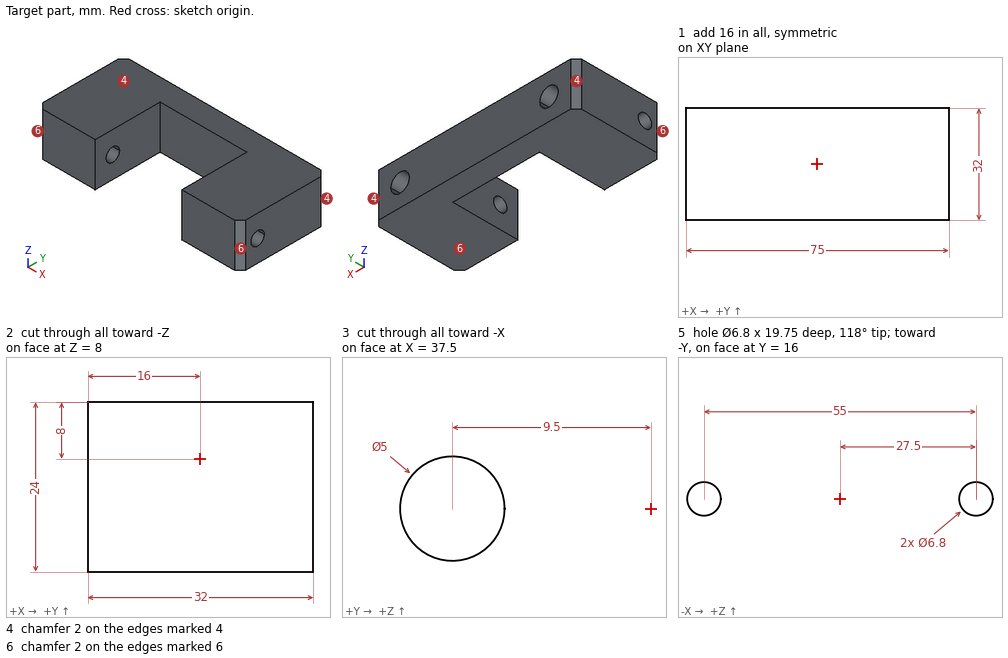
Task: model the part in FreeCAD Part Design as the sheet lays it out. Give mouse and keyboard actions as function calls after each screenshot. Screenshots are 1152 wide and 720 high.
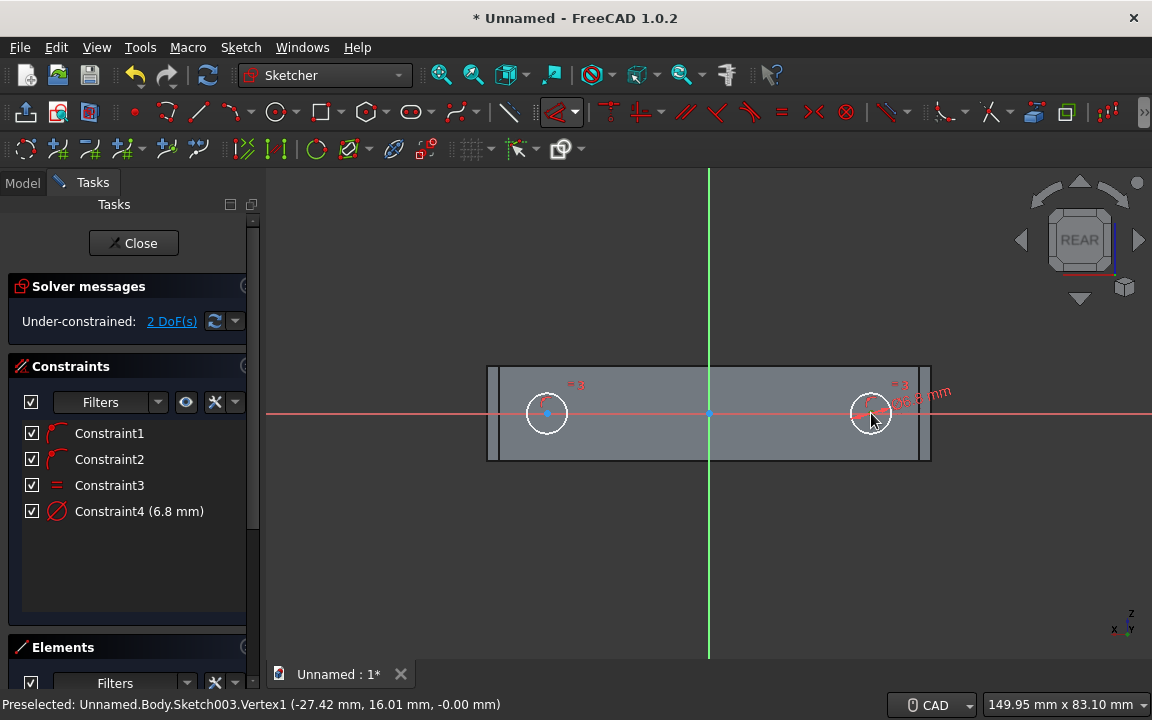
click(547, 413)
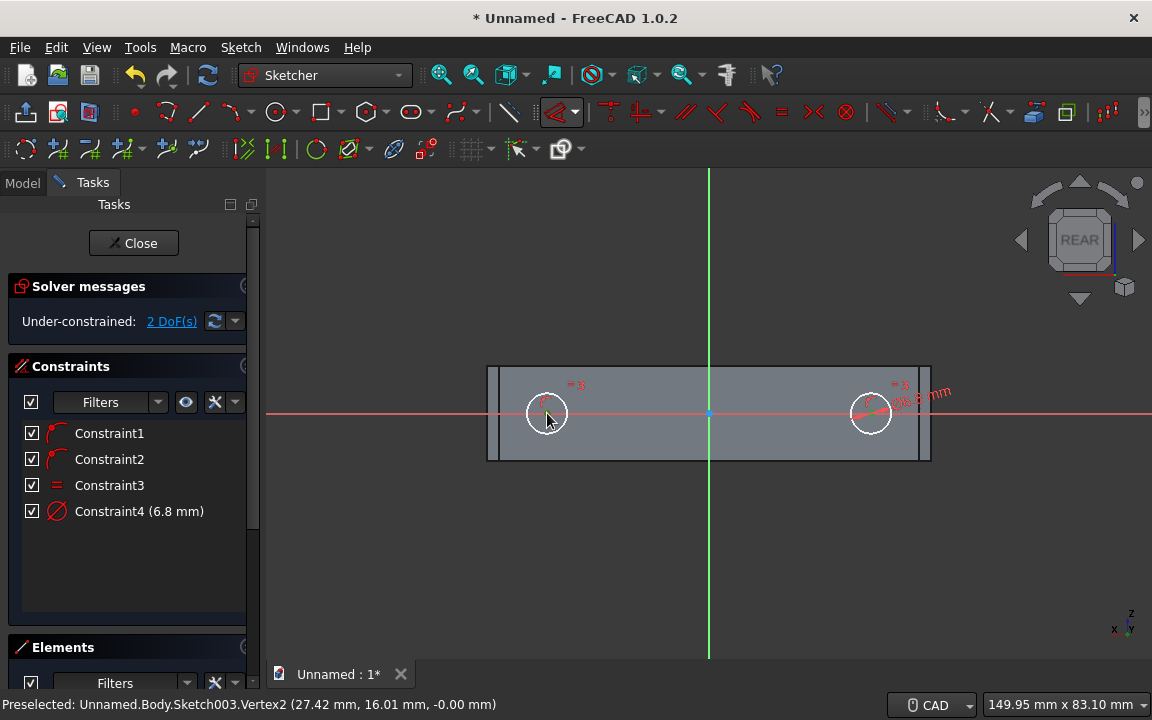
key(l)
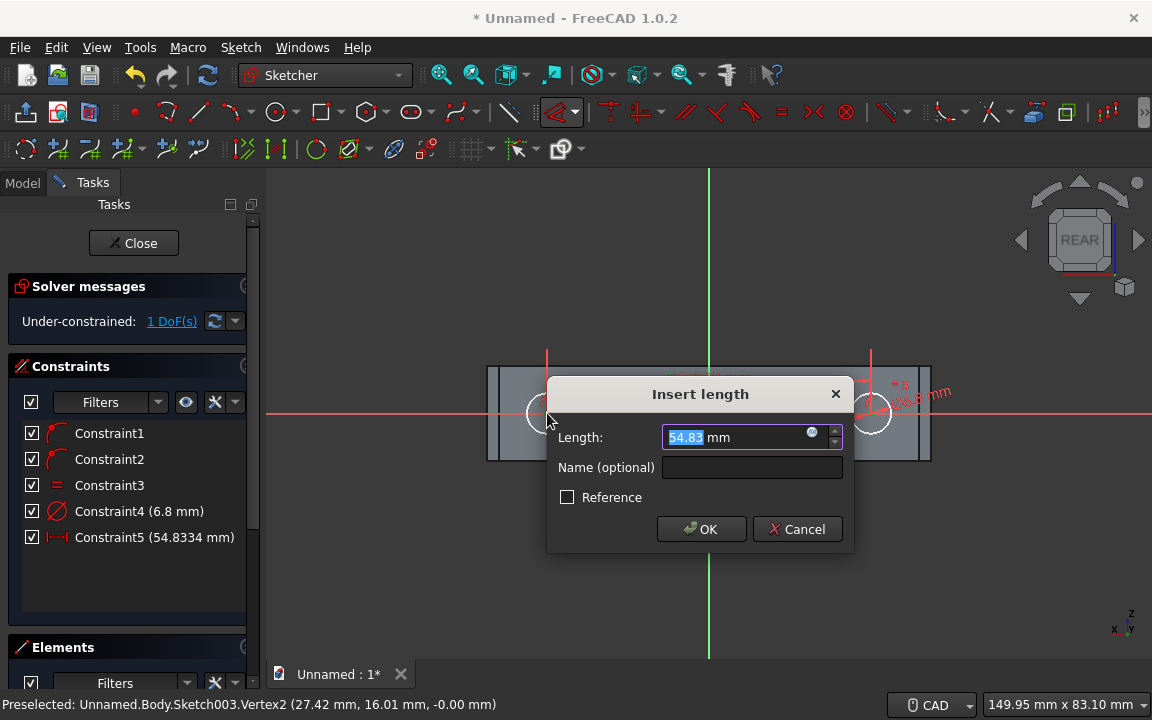
text(55)
key(Return)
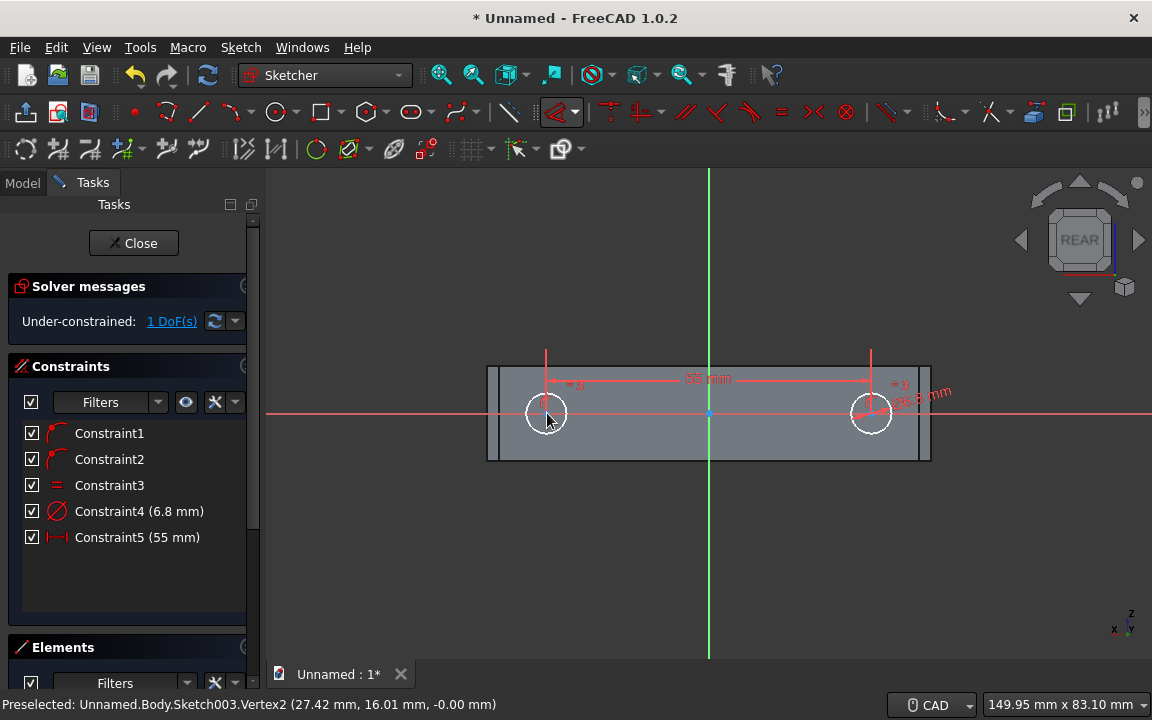
click(871, 413)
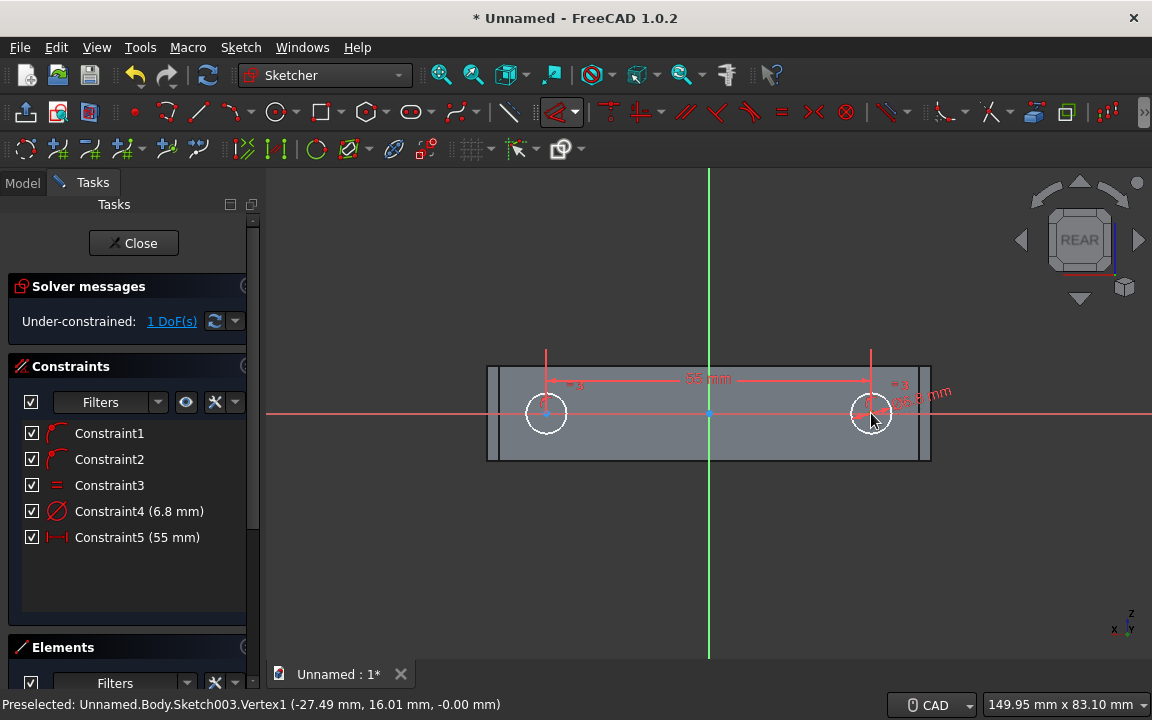
click(578, 112)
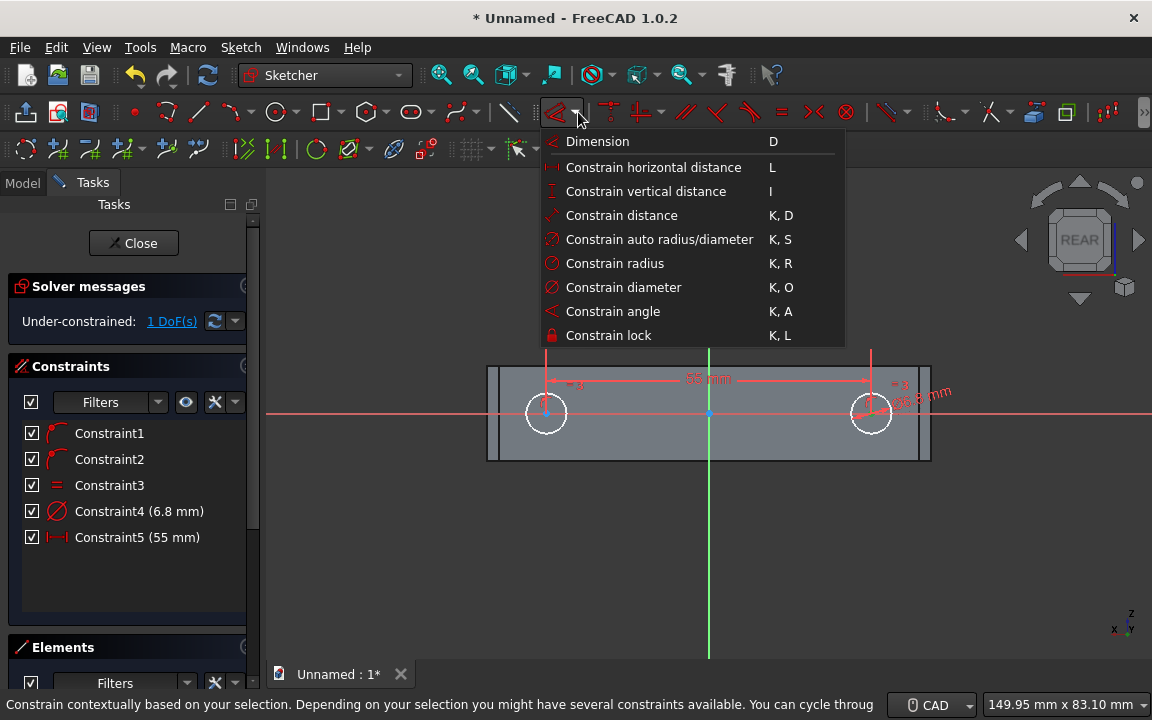
click(693, 167)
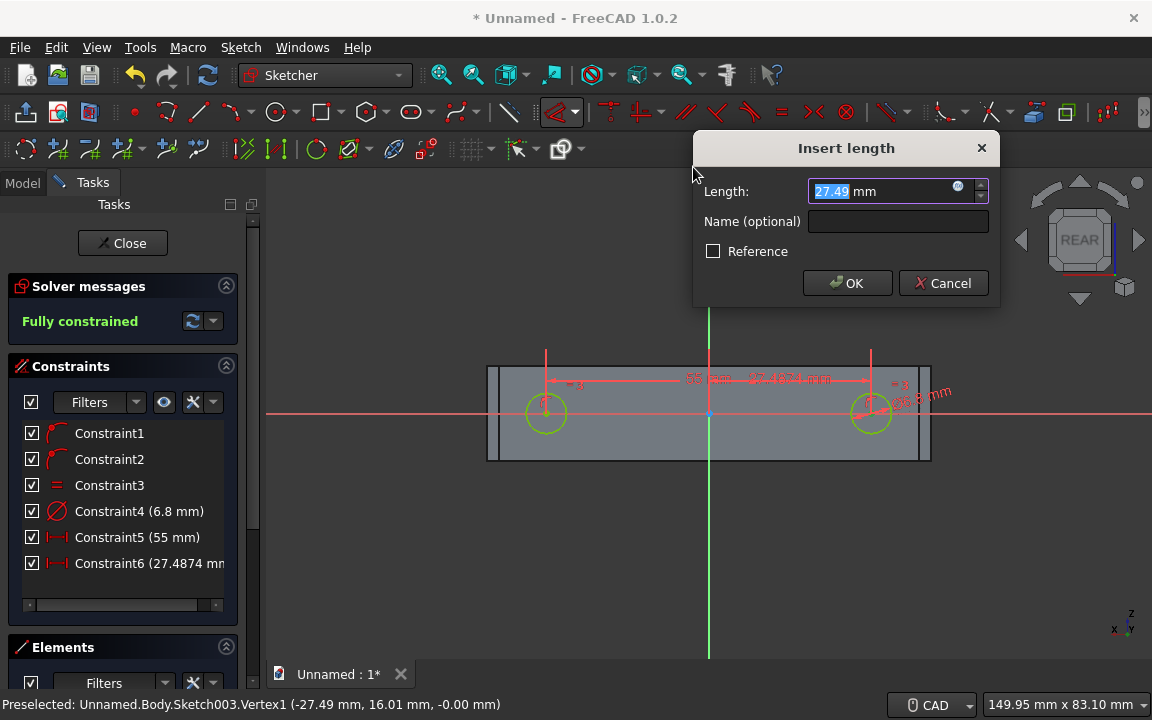
text(27.5)
key(Return)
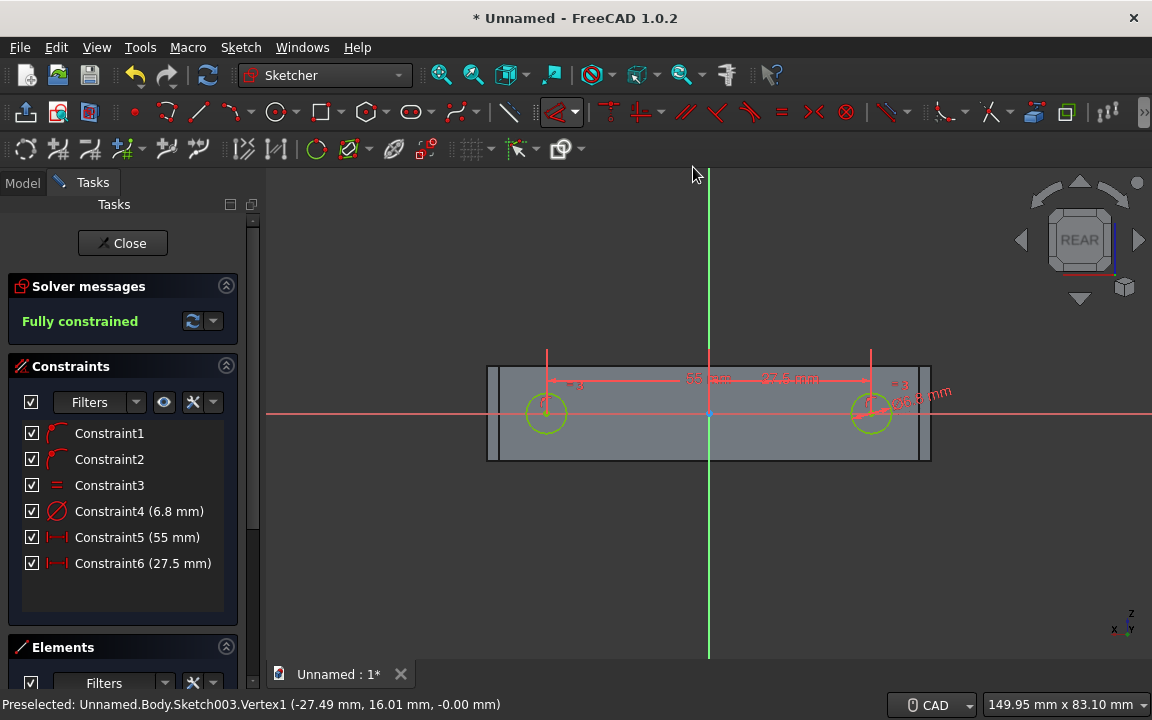
click(123, 243)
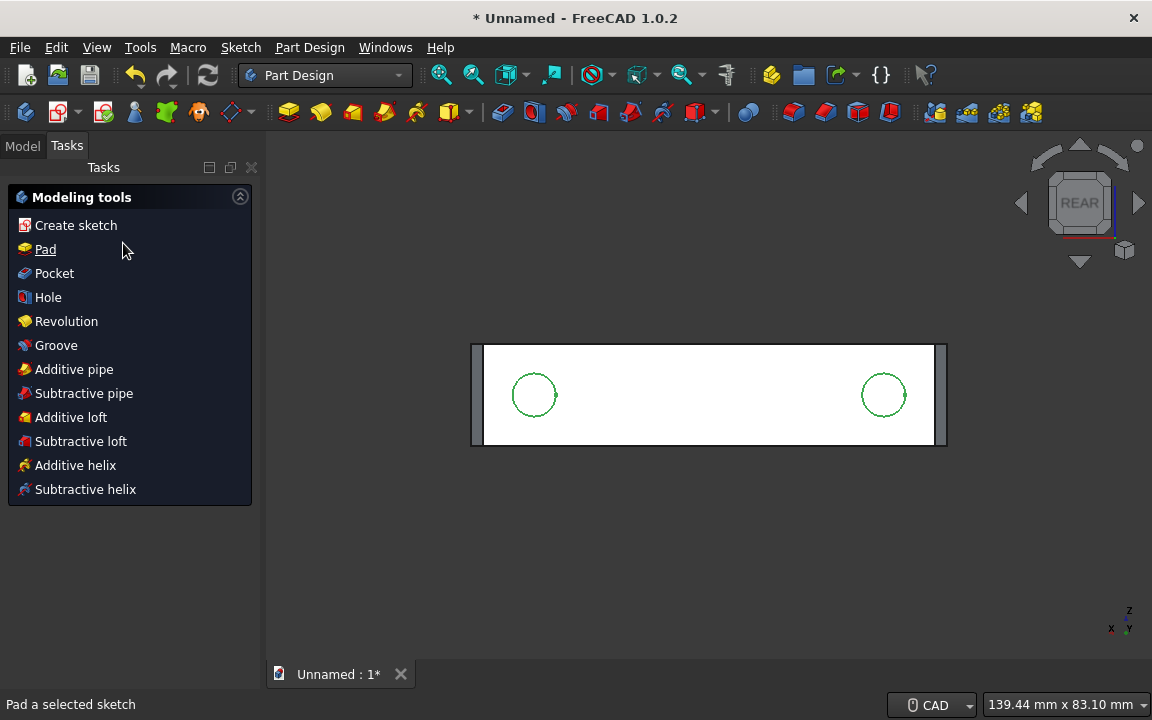
click(536, 112)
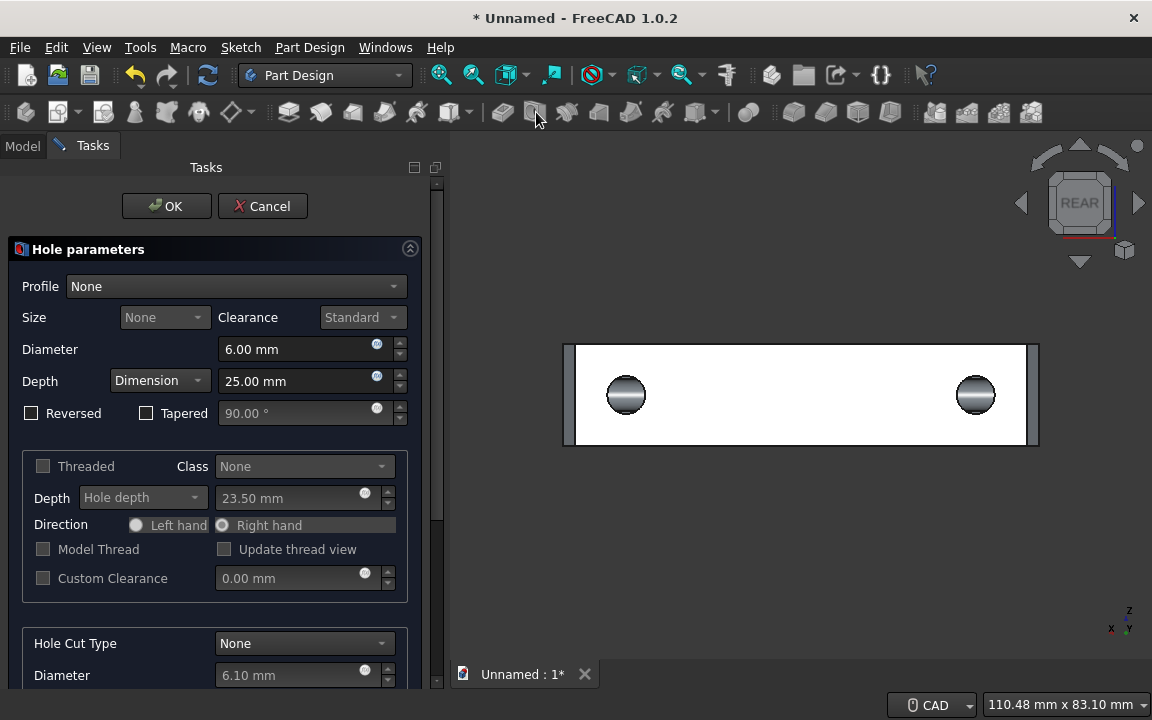
triple_click(305, 349)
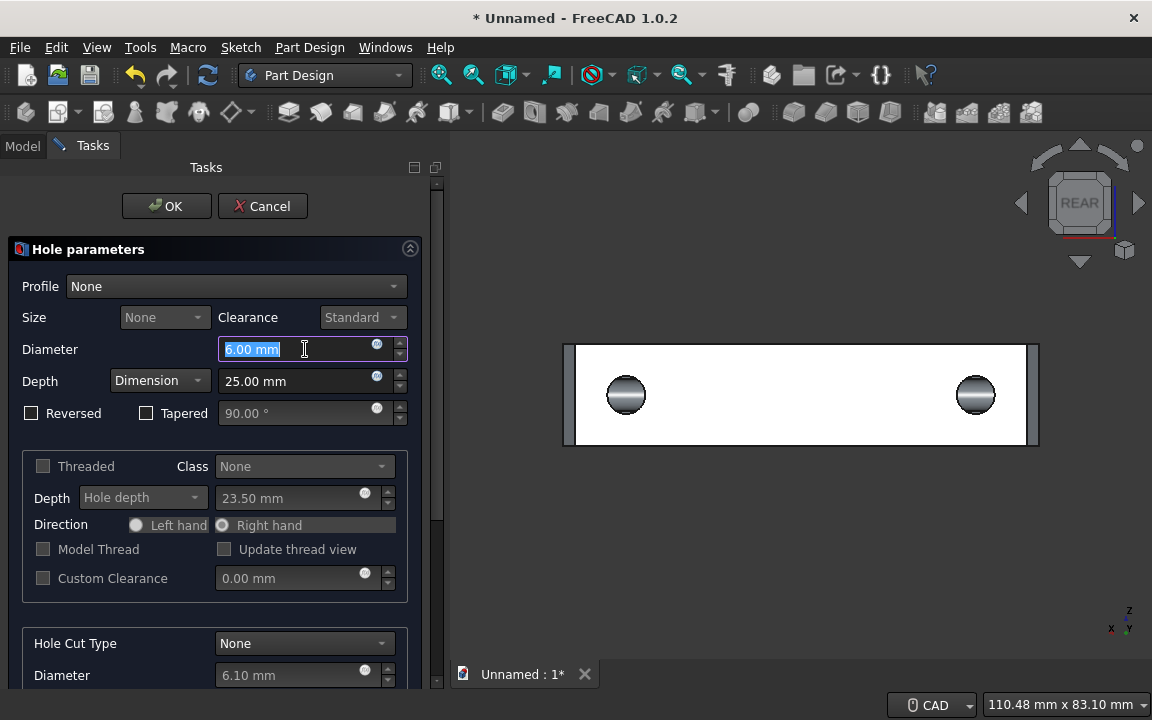
text(6.8)
key(Tab)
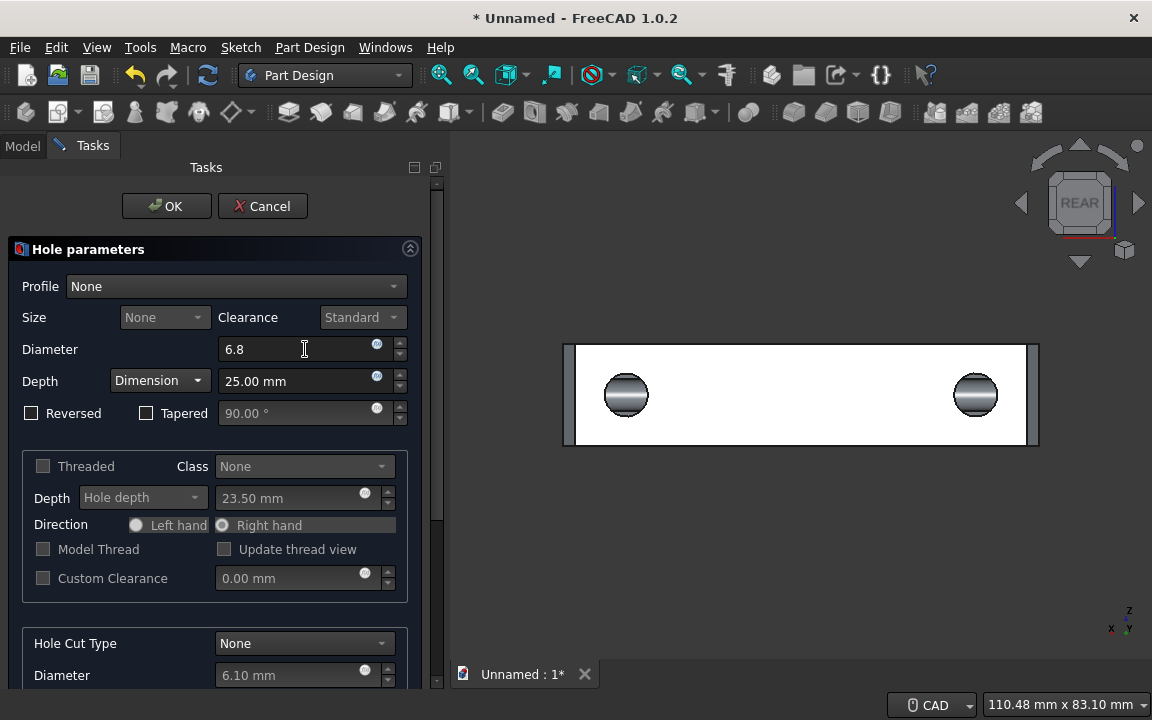
triple_click(305, 381)